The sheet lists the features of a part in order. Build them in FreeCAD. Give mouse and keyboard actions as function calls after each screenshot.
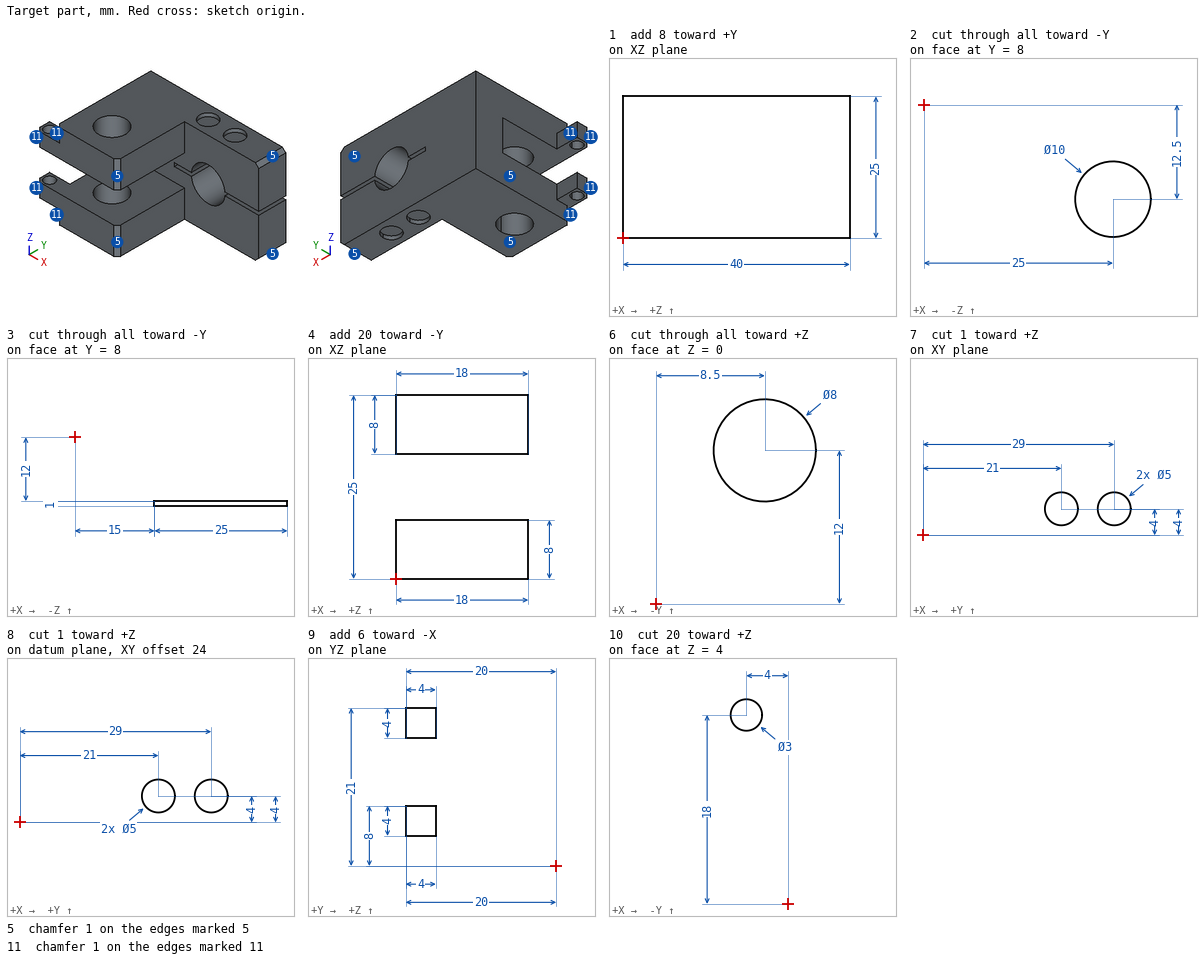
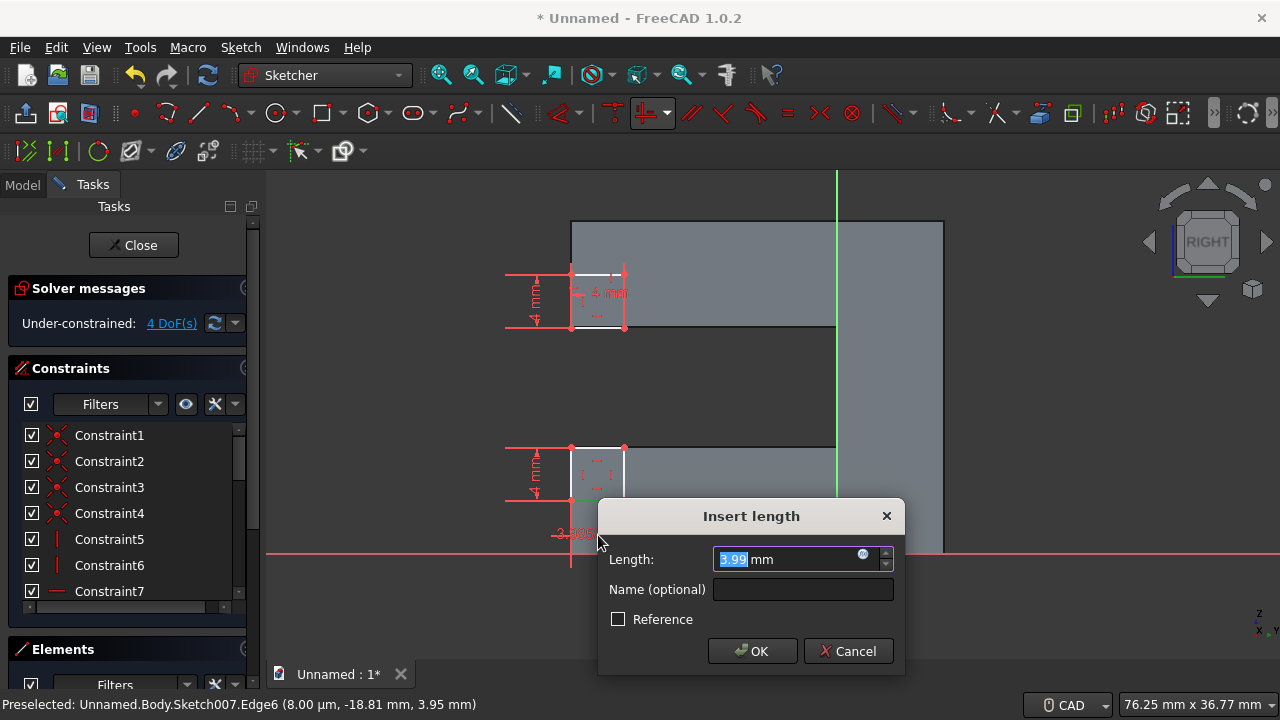
text(4)
key(Return)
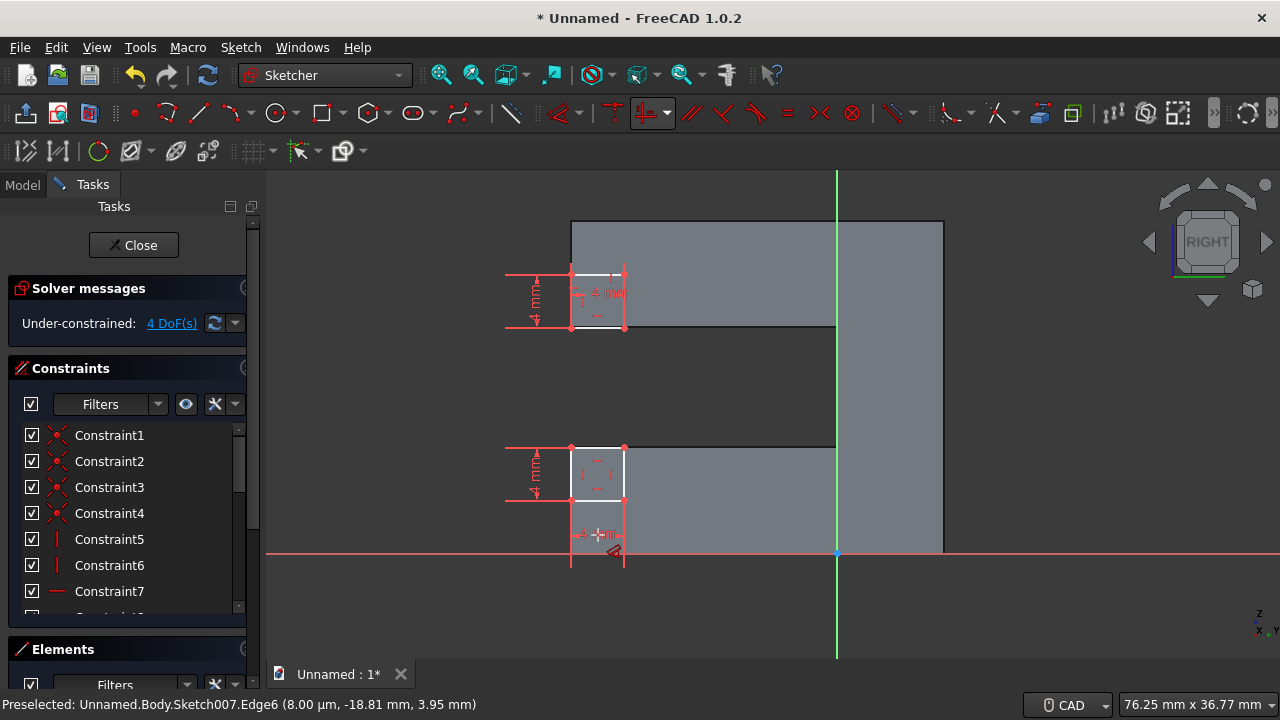
click(571, 448)
click(537, 501)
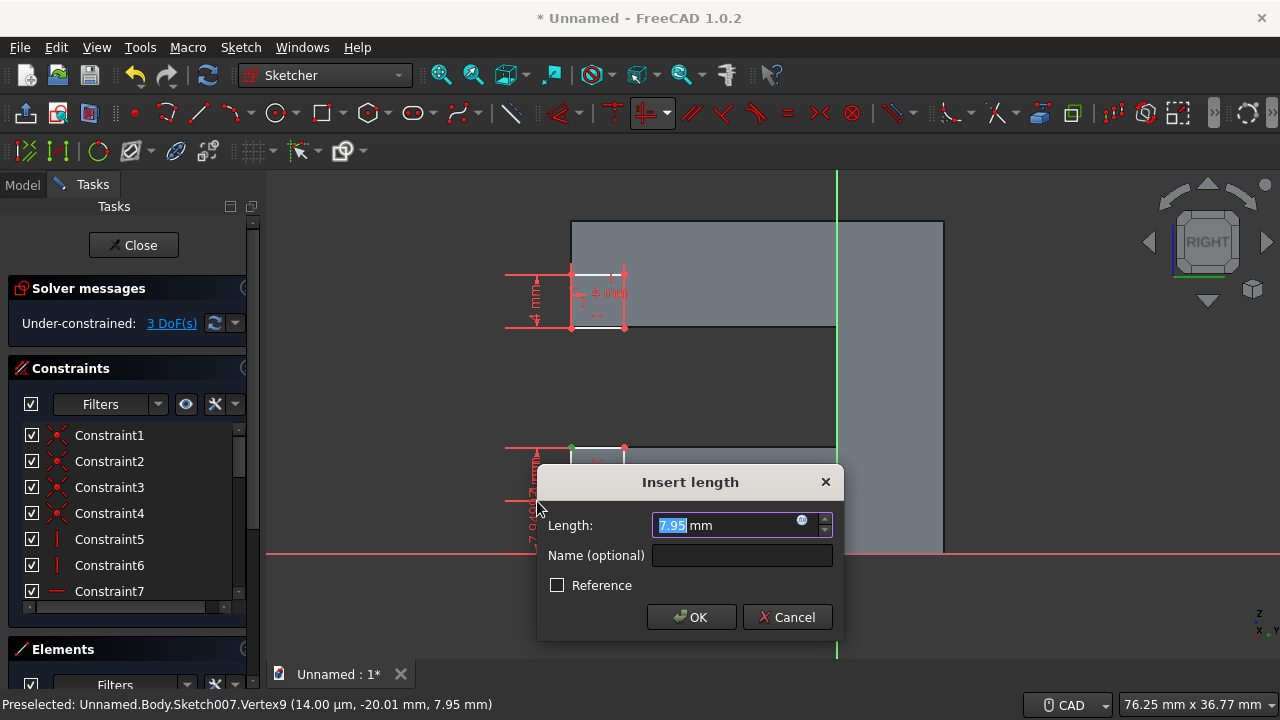
text(8)
key(Return)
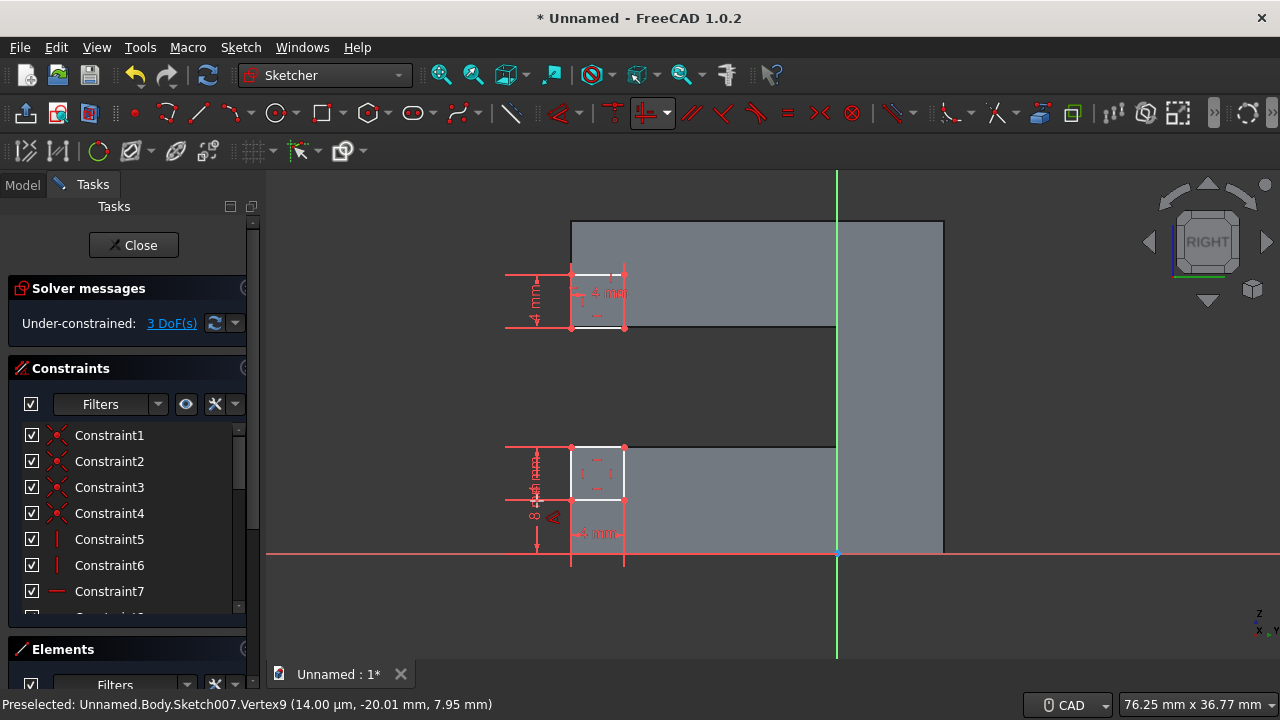
click(571, 275)
click(704, 588)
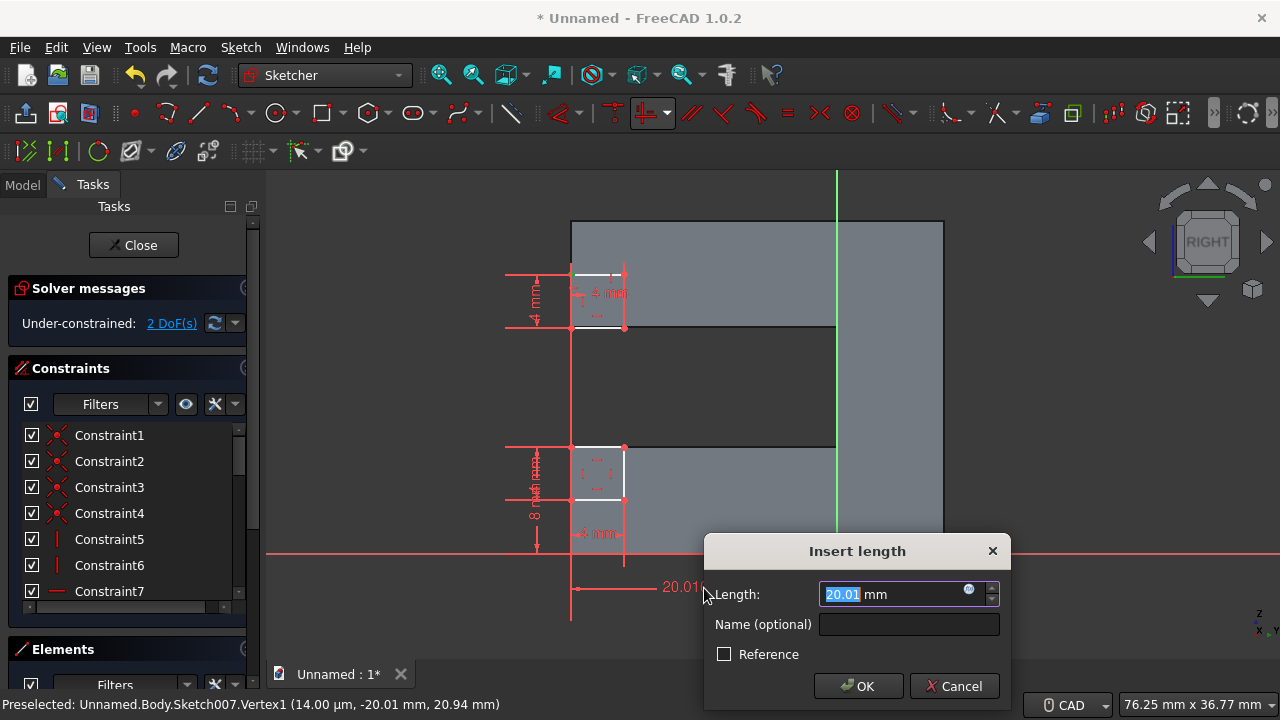
text(20)
key(Return)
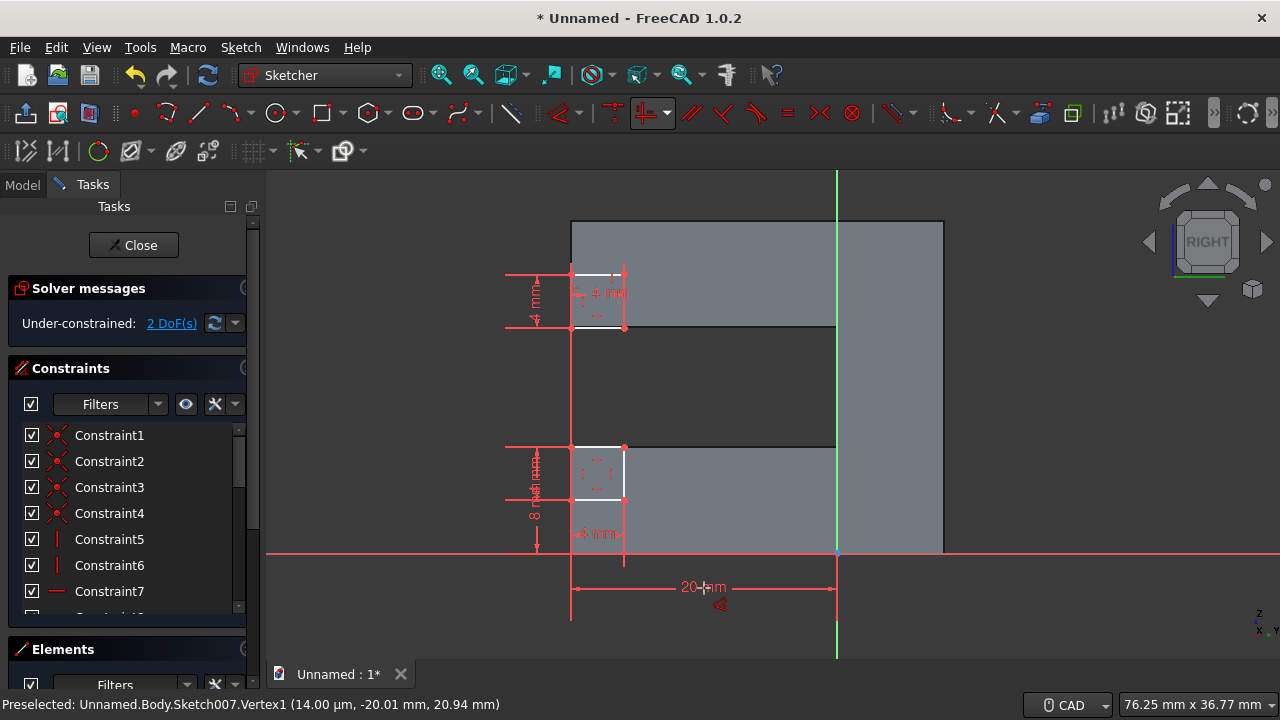
click(571, 275)
click(871, 414)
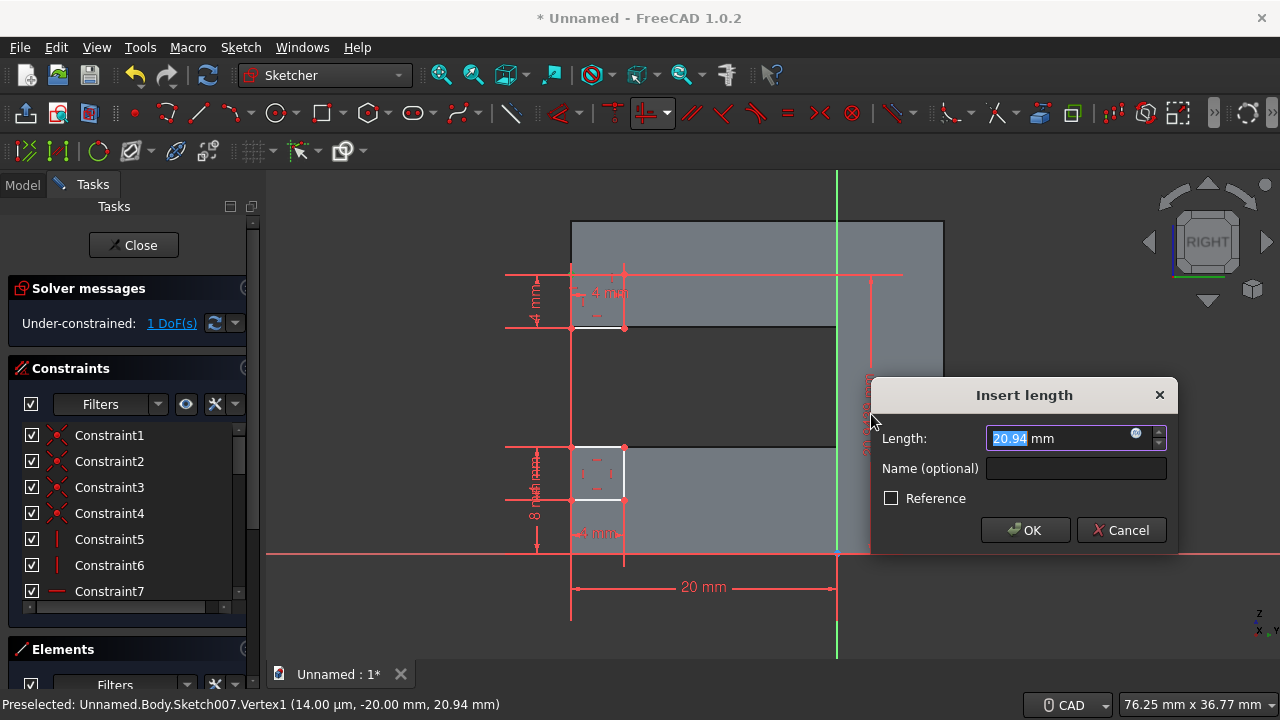
text(21)
key(Return)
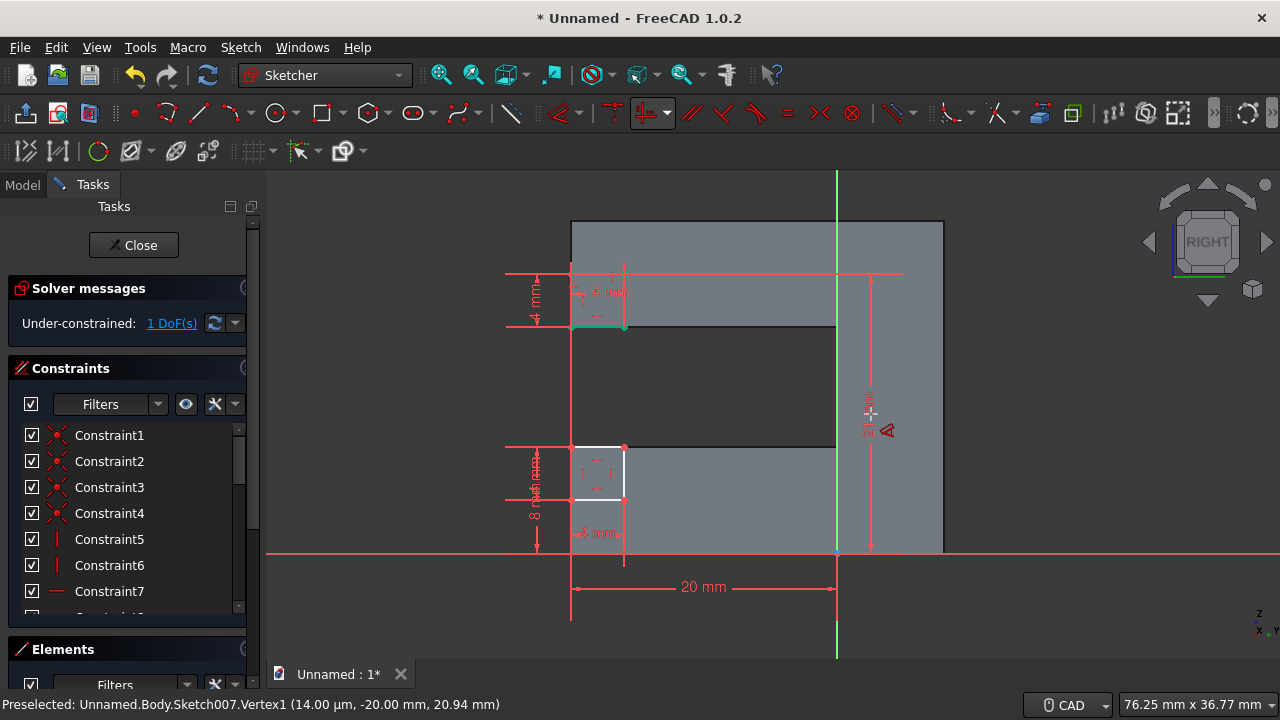
click(571, 447)
click(611, 588)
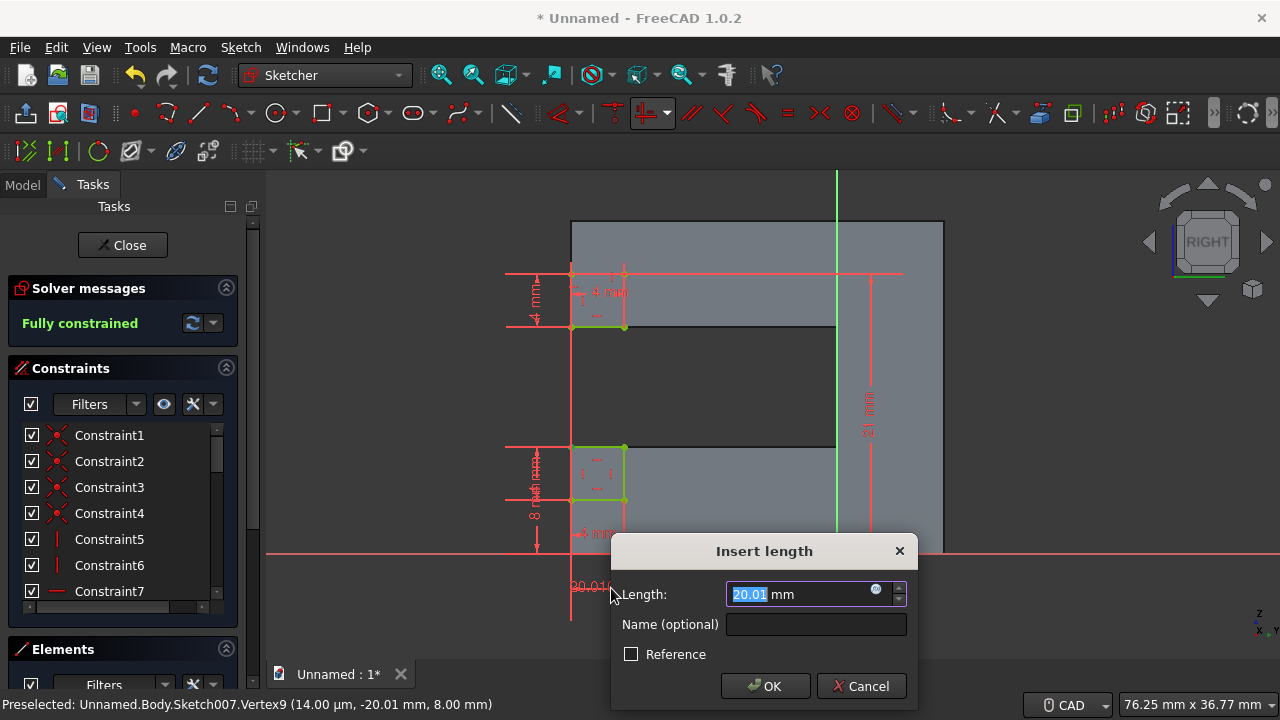
text(20)
key(Return)
key(Escape)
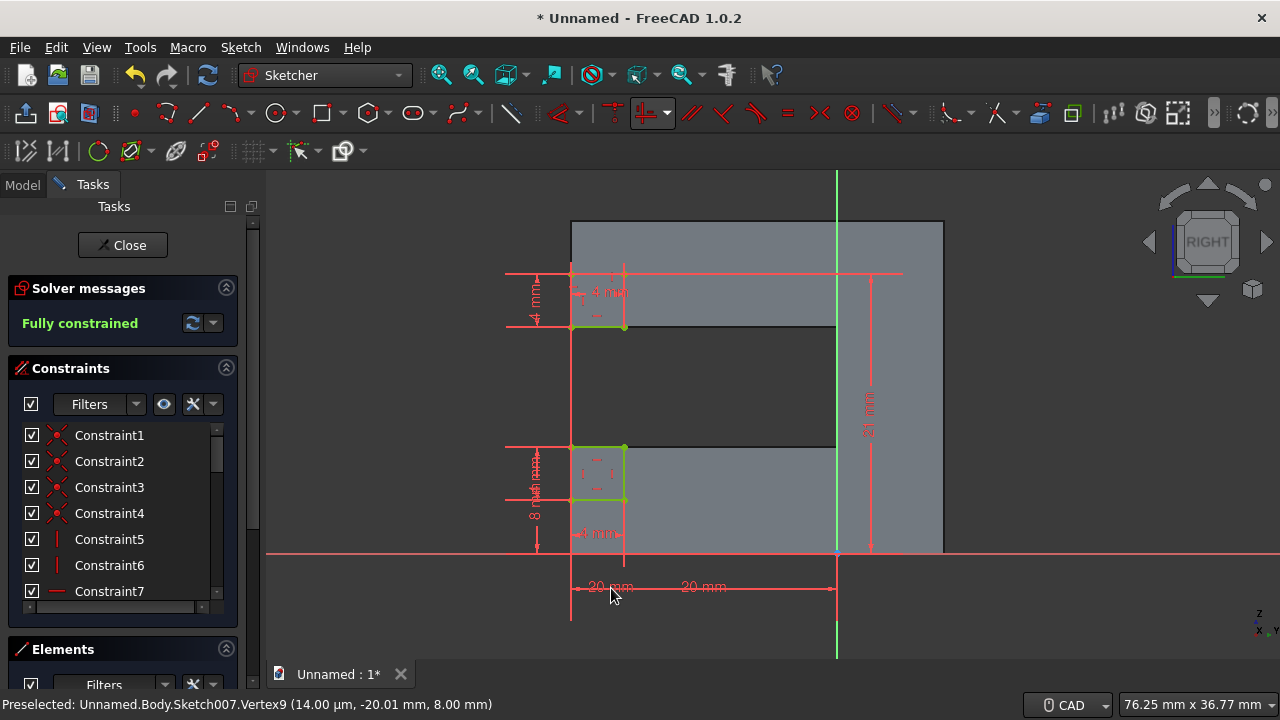
click(123, 245)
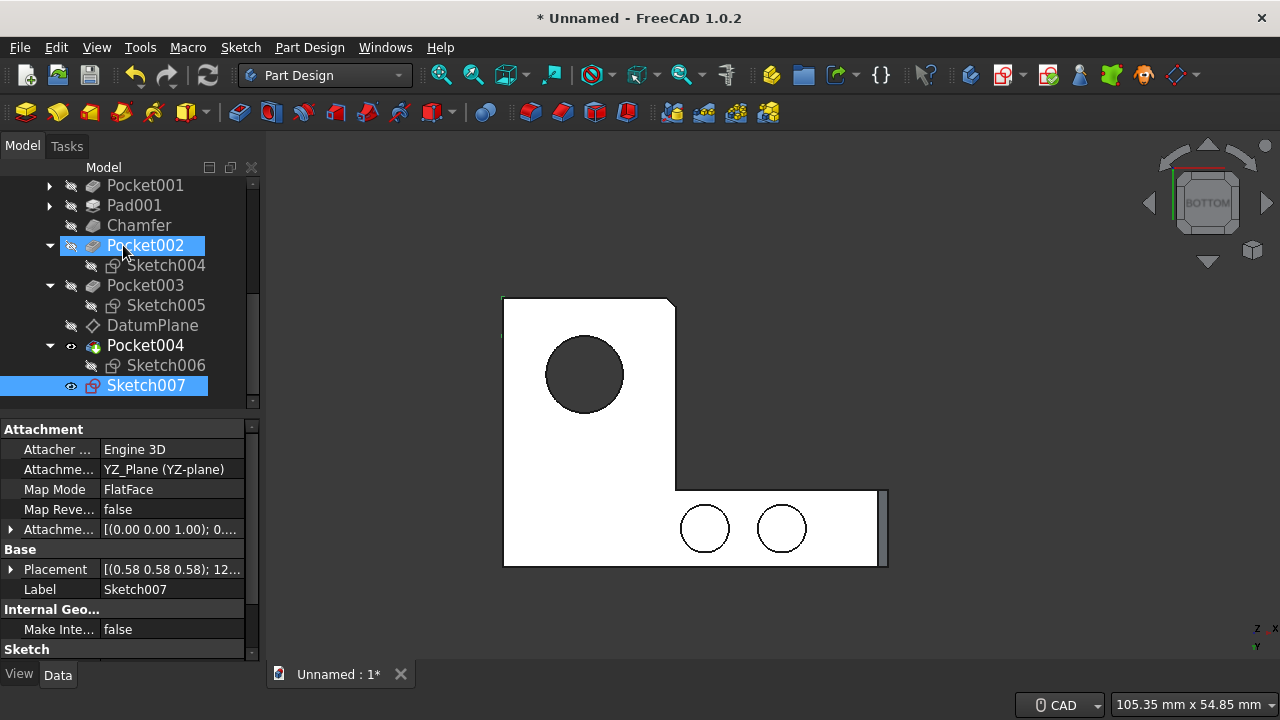
click(26, 112)